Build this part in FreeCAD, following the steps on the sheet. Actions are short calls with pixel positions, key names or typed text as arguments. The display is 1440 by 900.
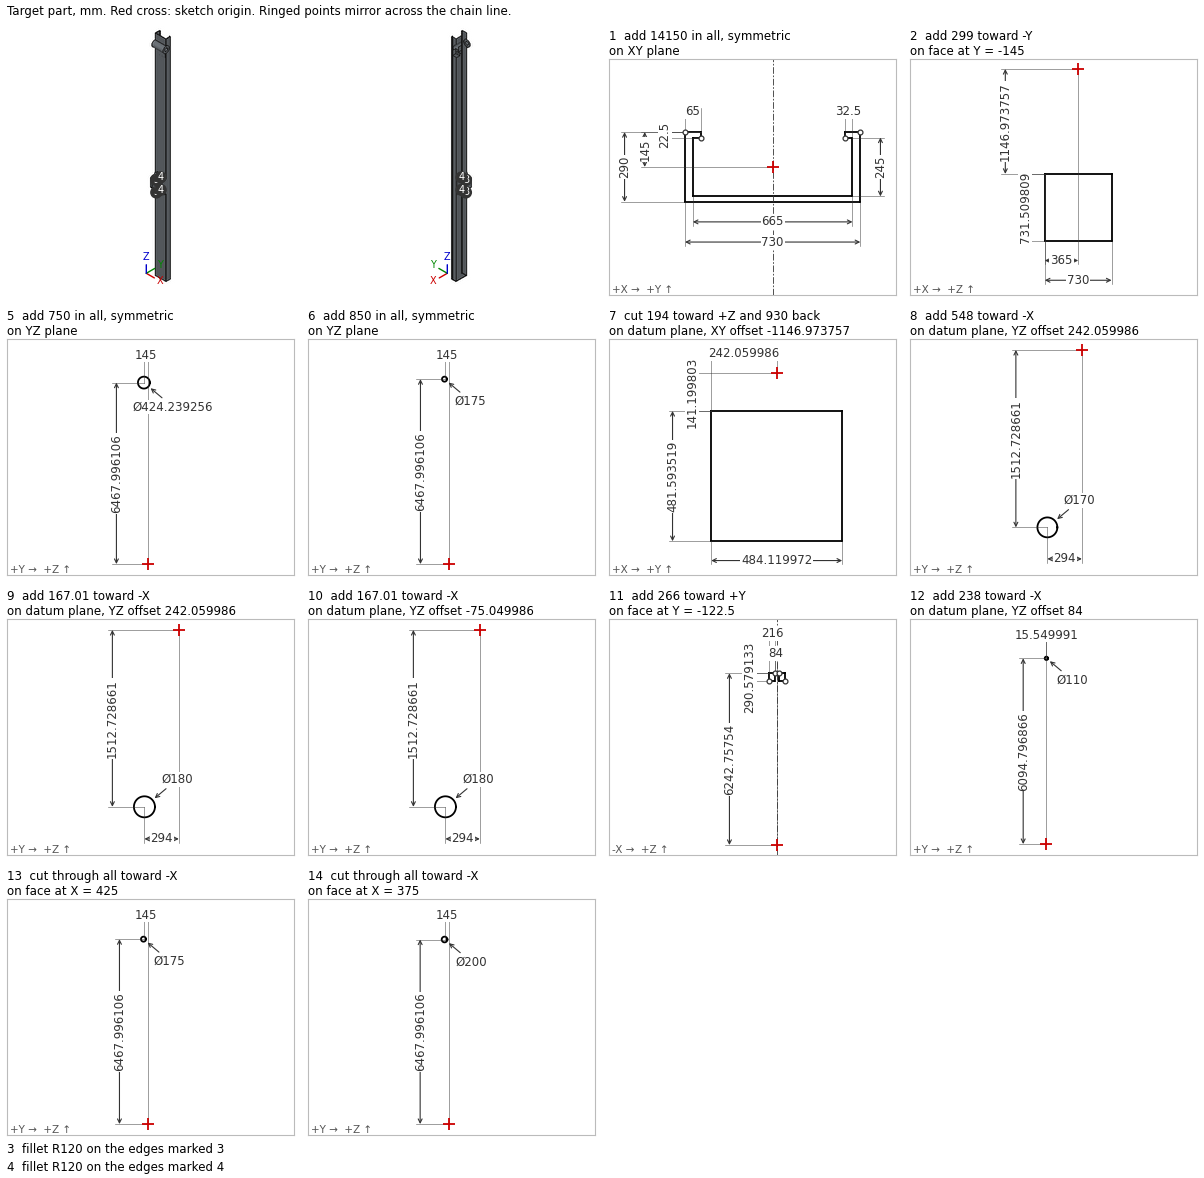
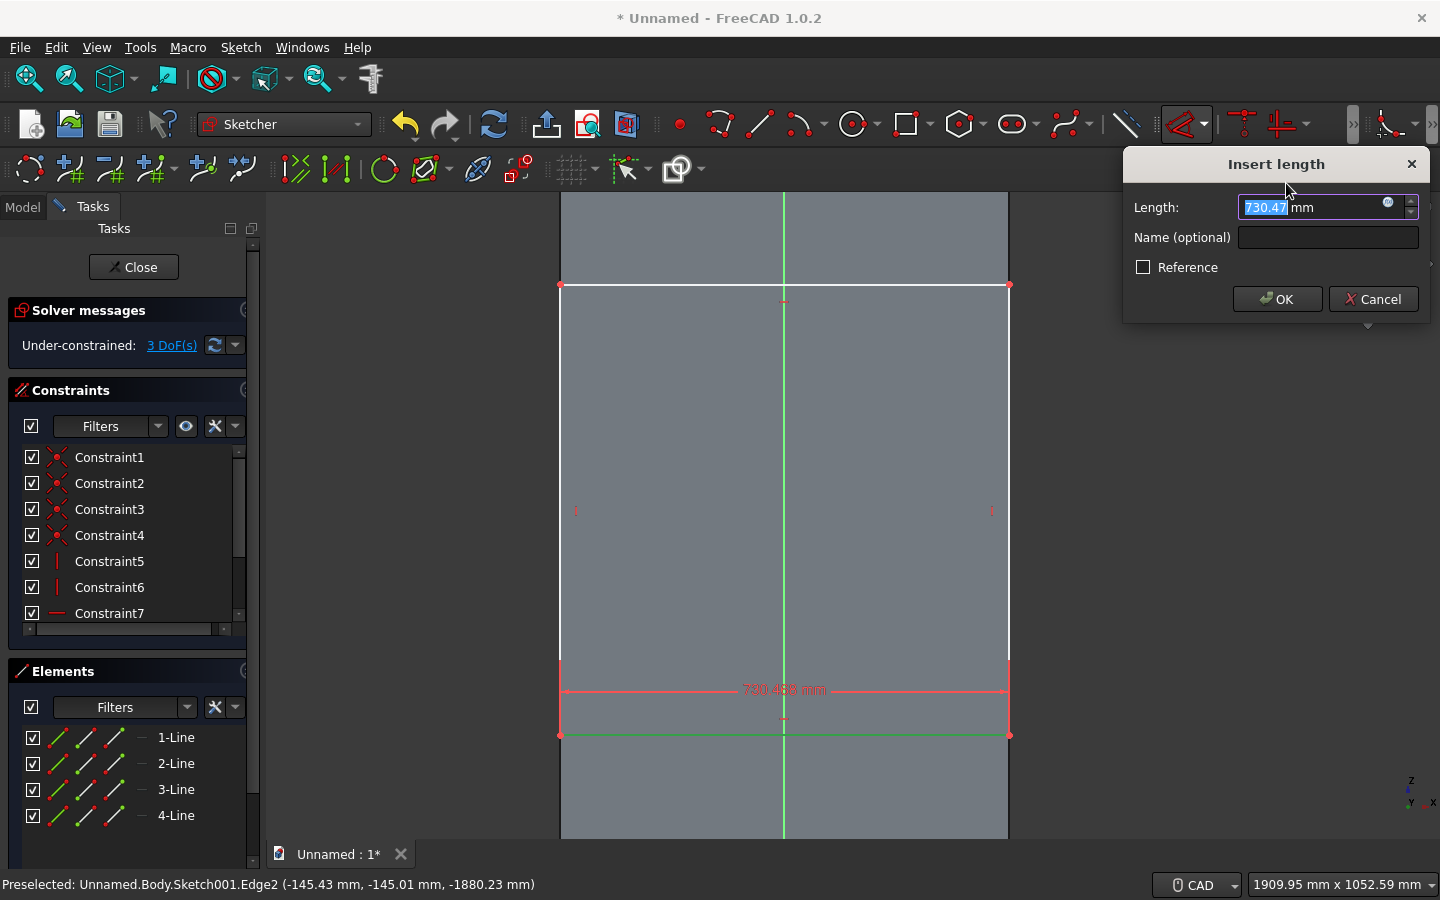
text(730)
key(Return)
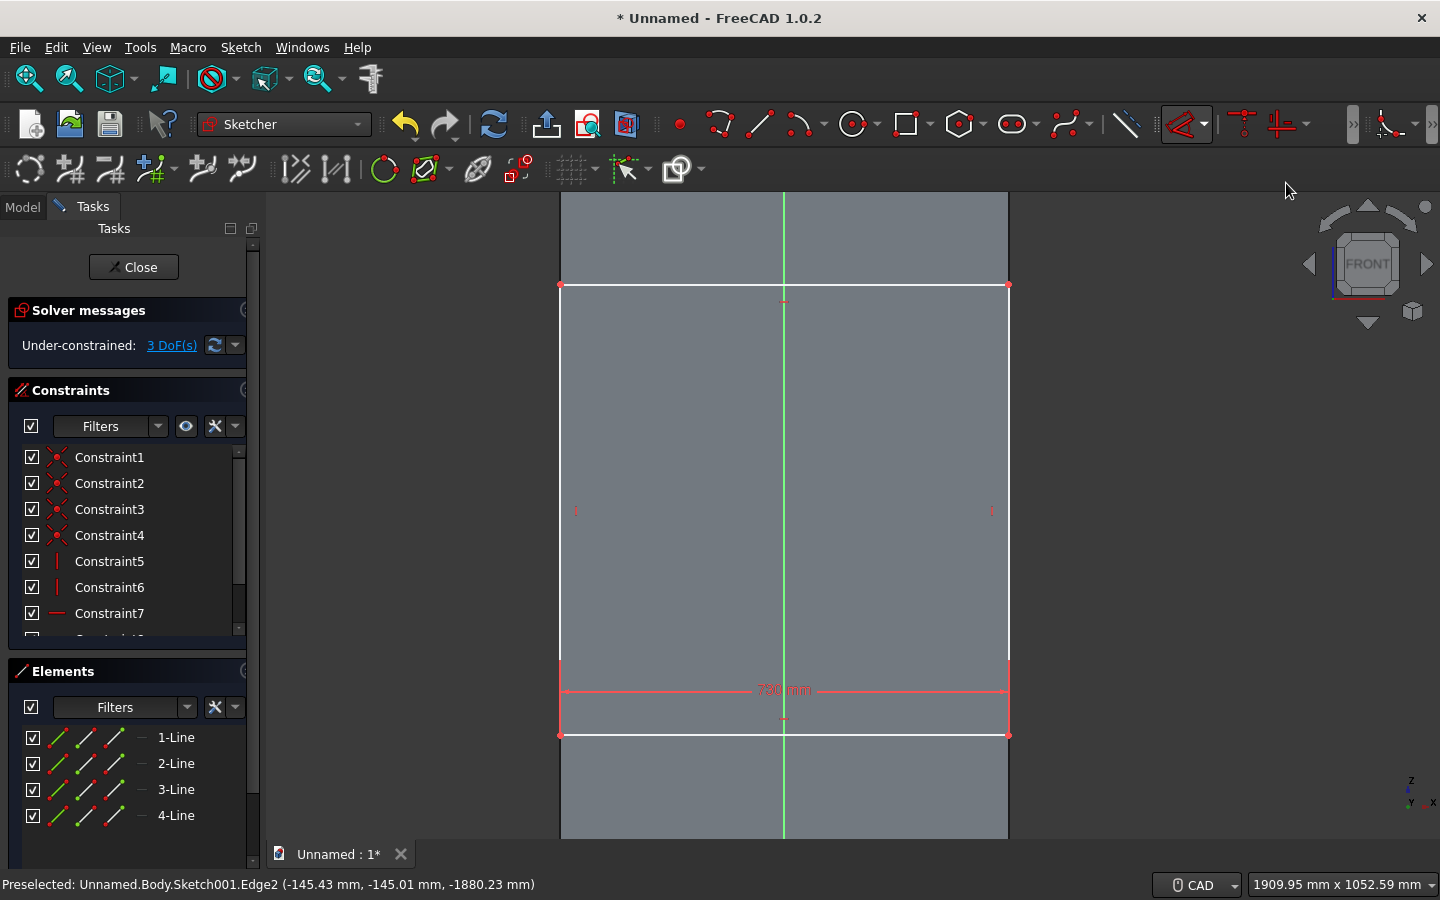
click(560, 285)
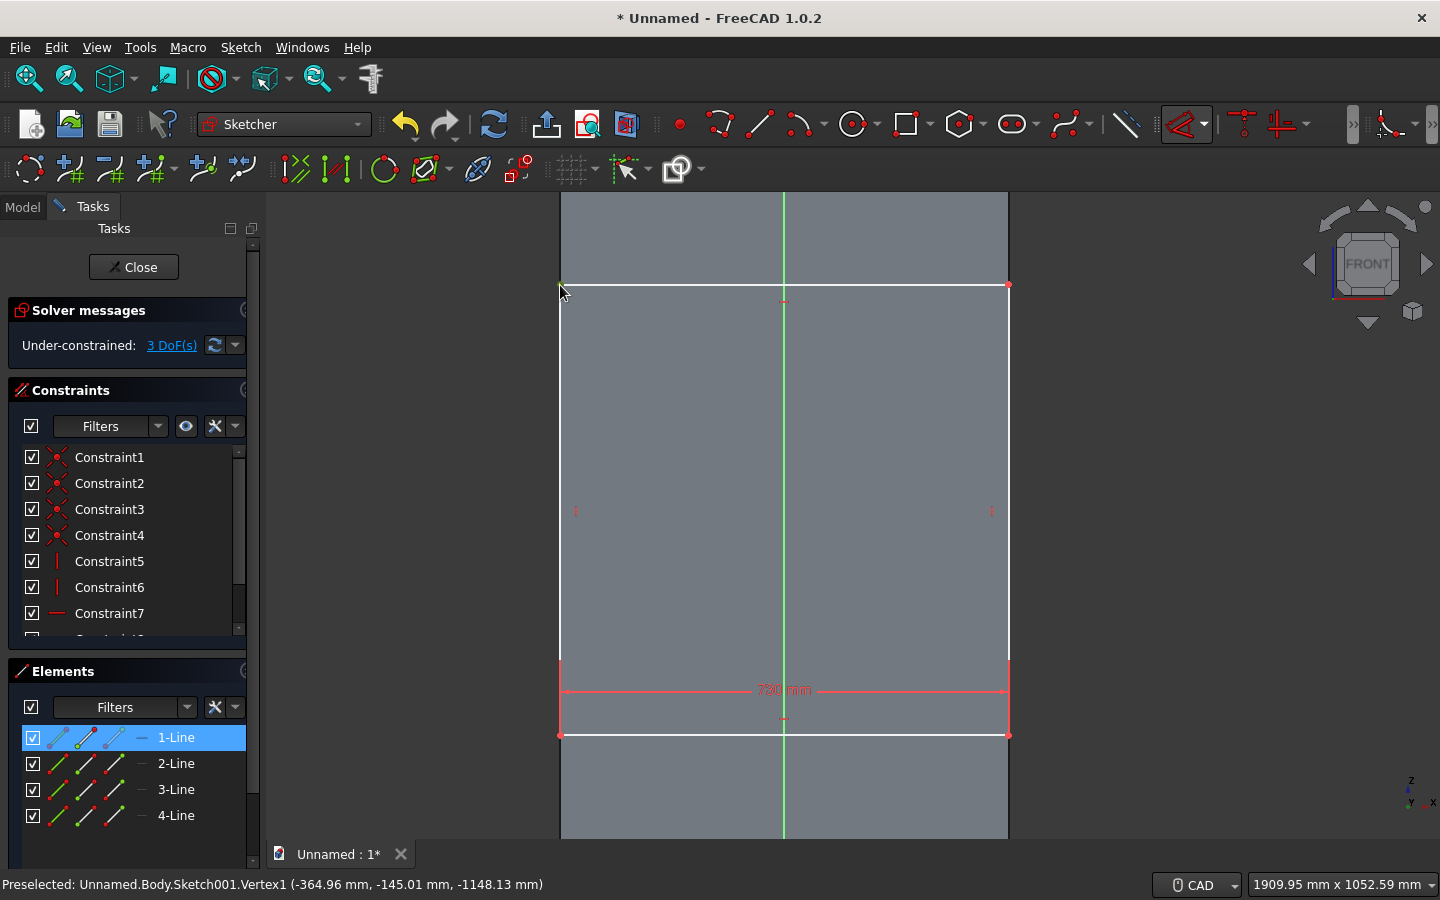
key(l)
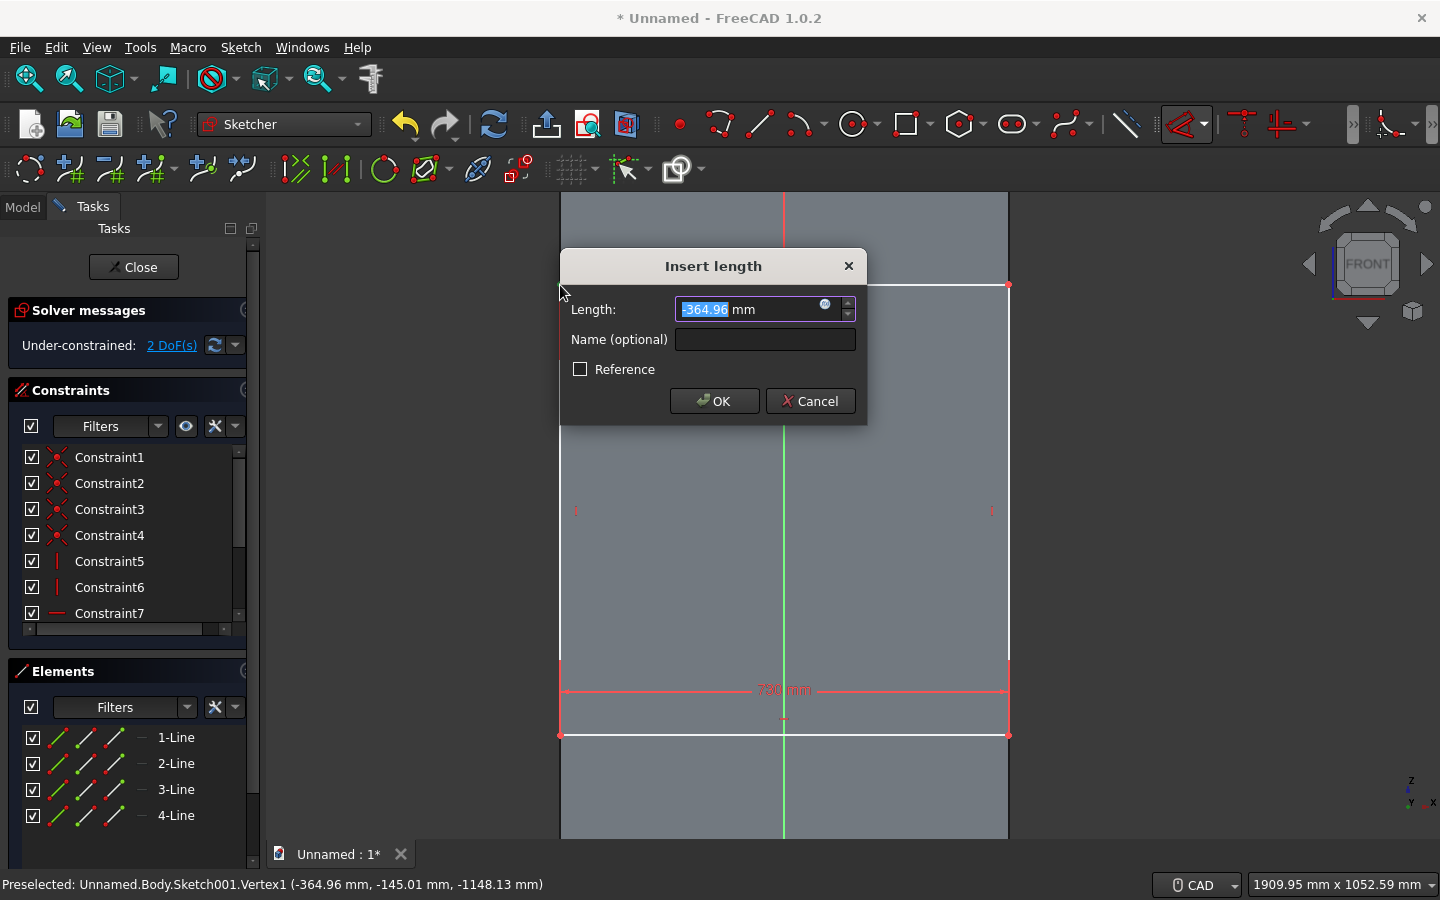
text(-365)
key(Return)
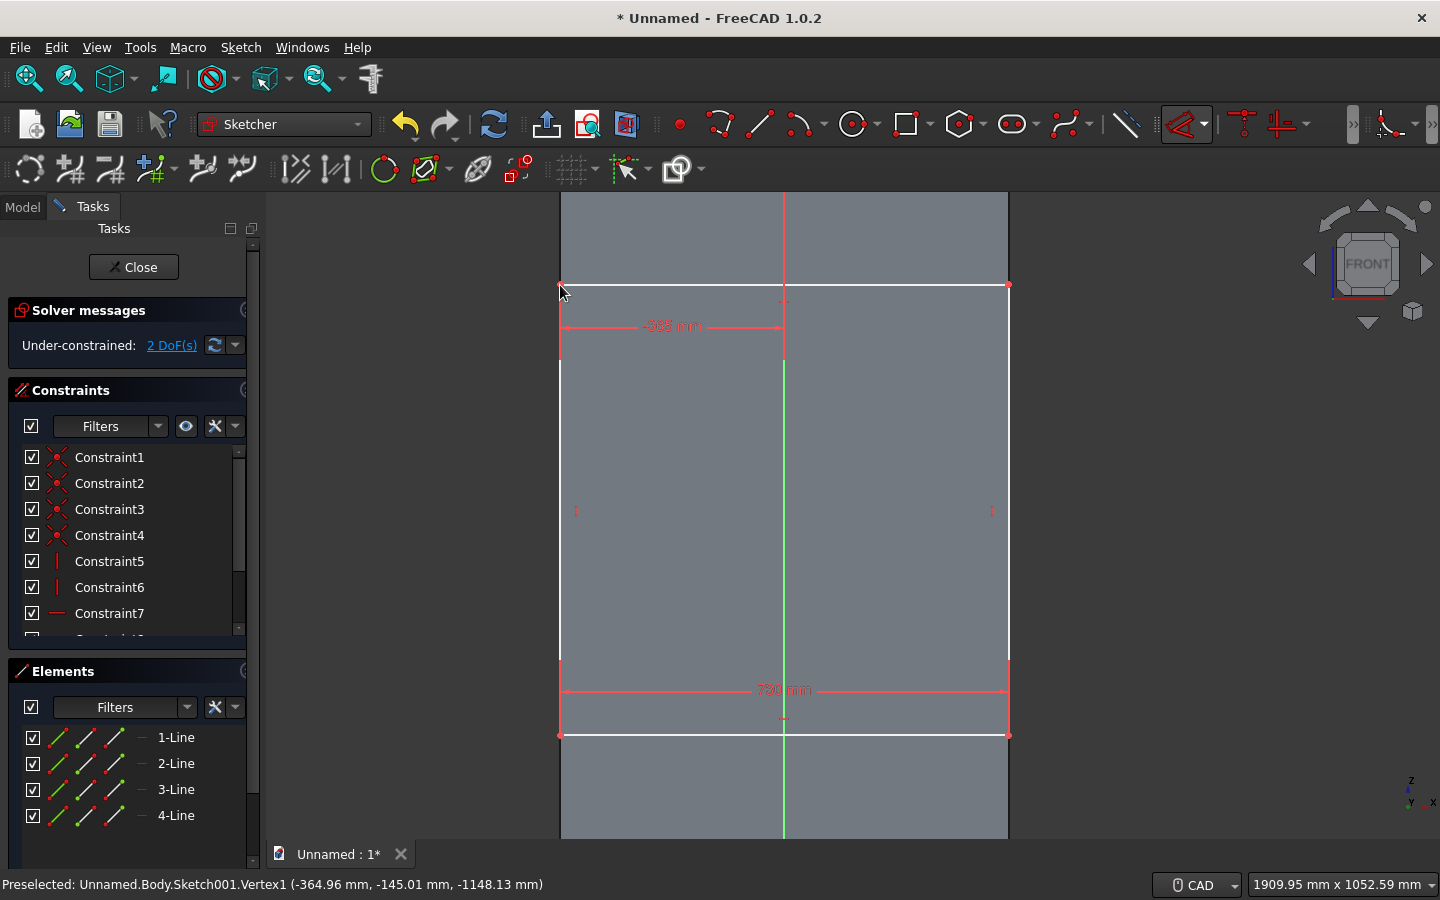
click(560, 420)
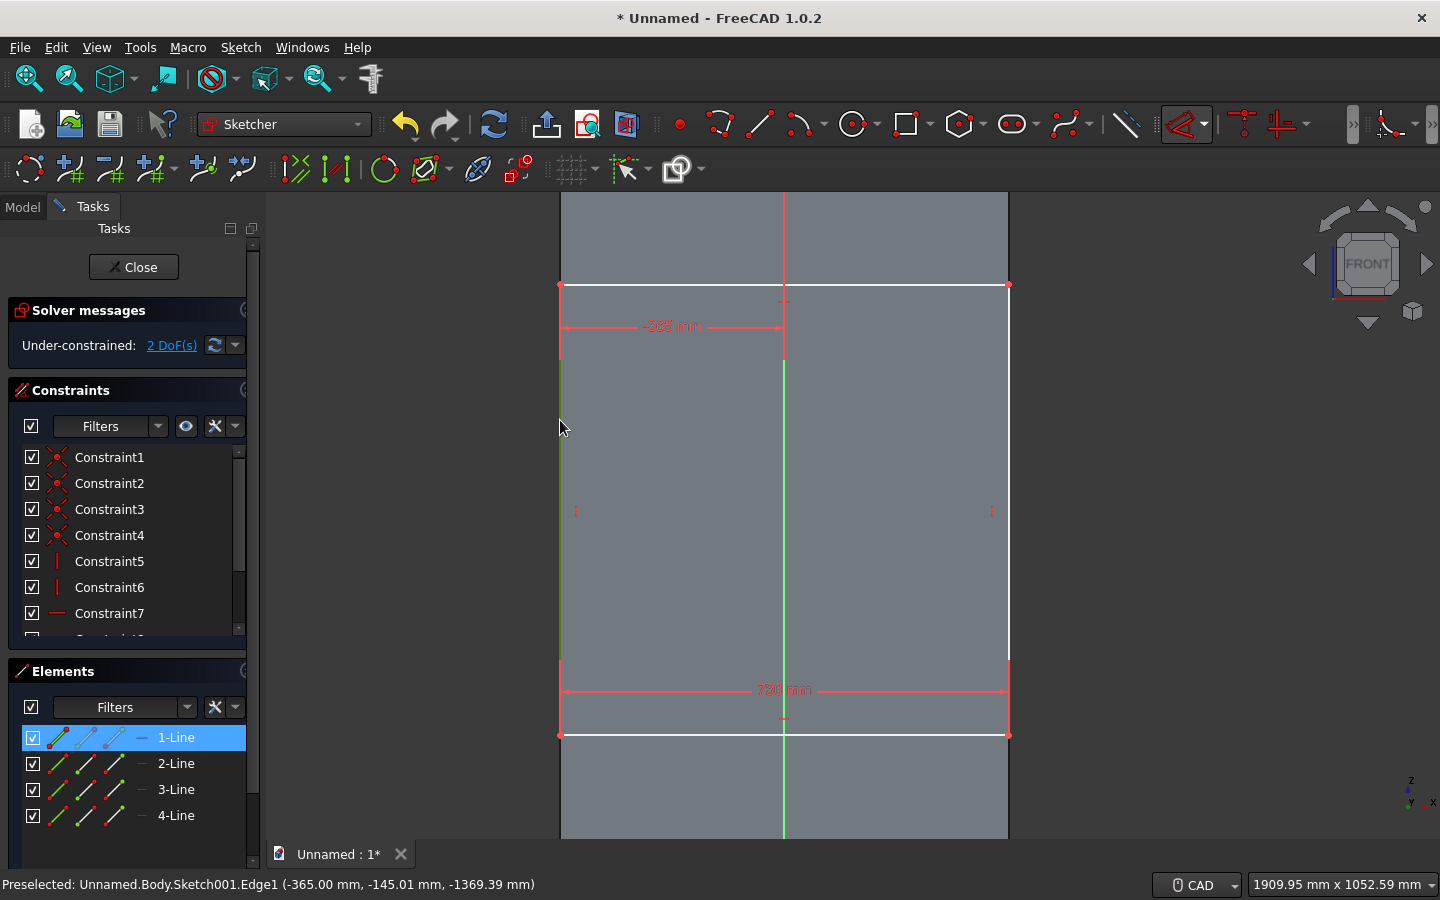
key(i)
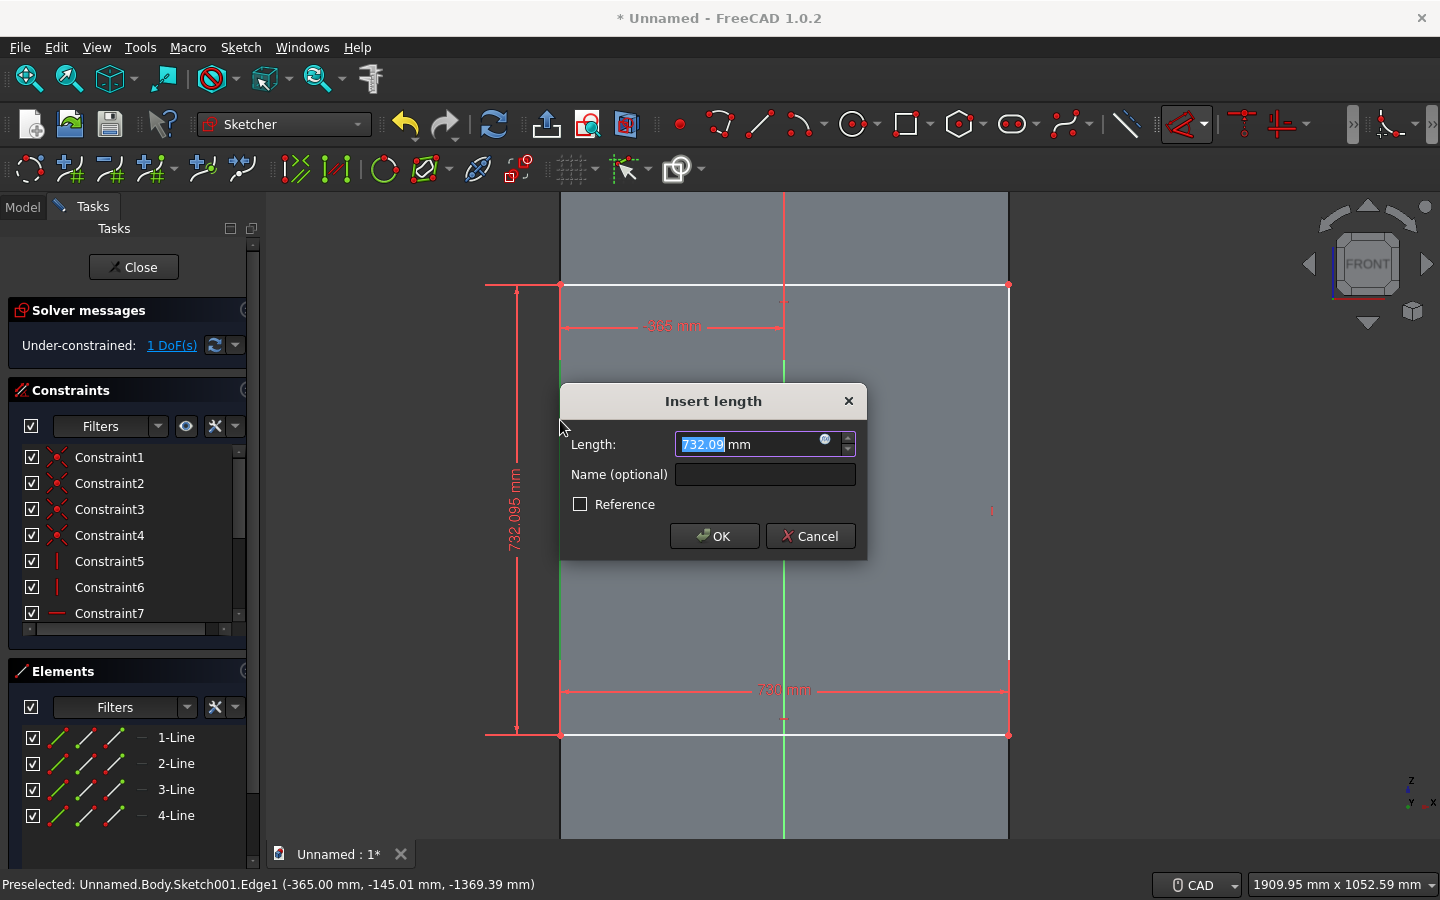
text(731.509809)
key(Return)